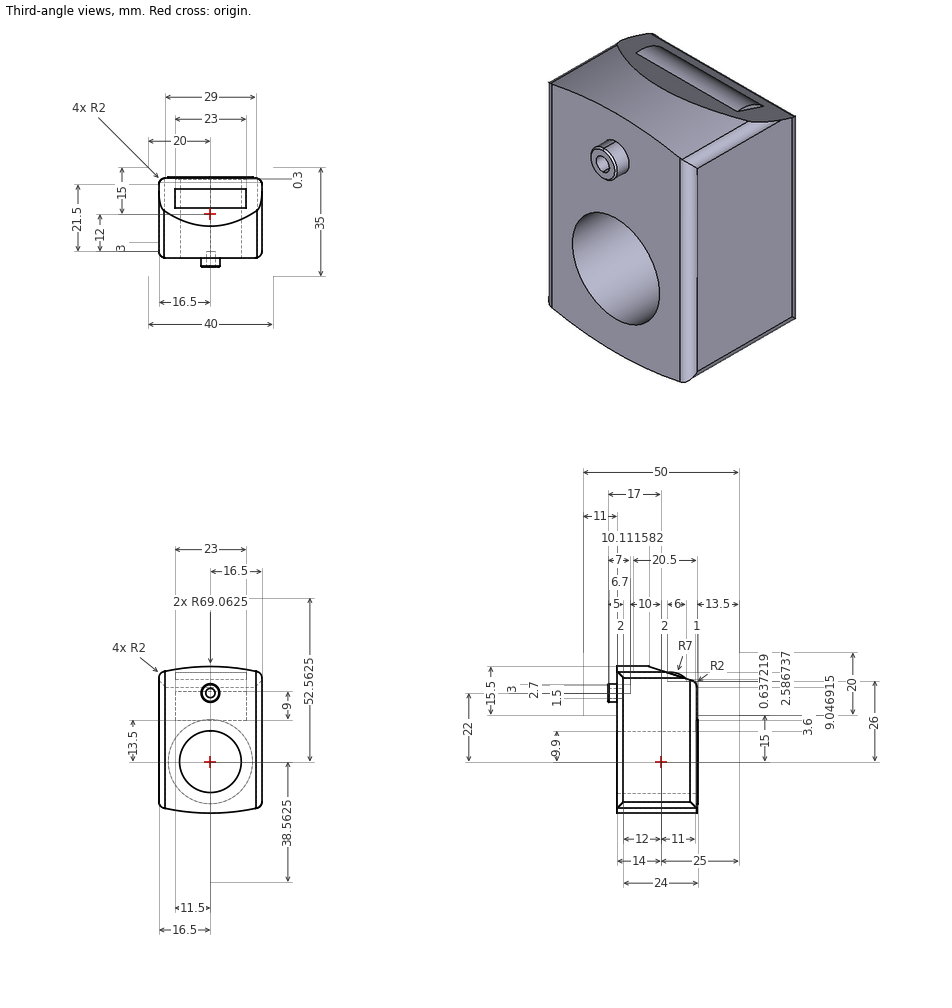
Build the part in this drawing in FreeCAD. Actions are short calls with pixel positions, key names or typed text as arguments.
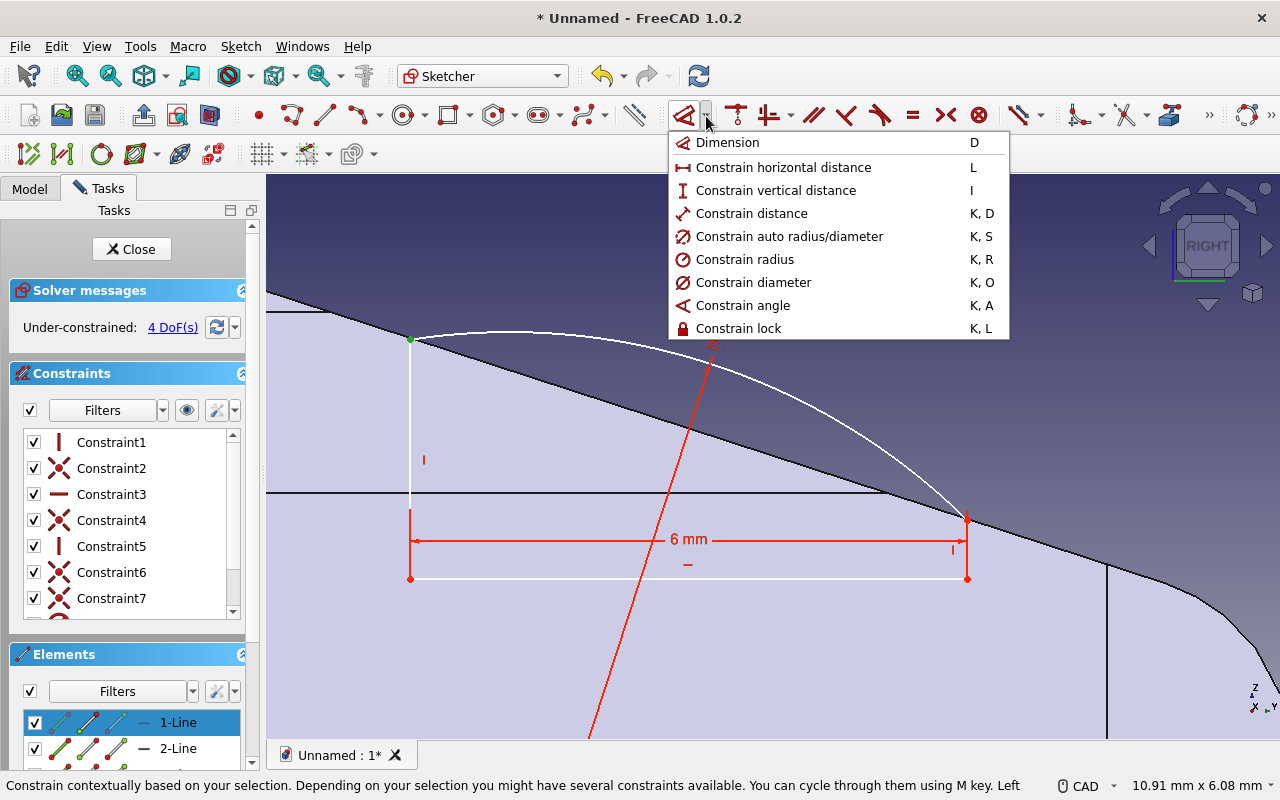
click(839, 168)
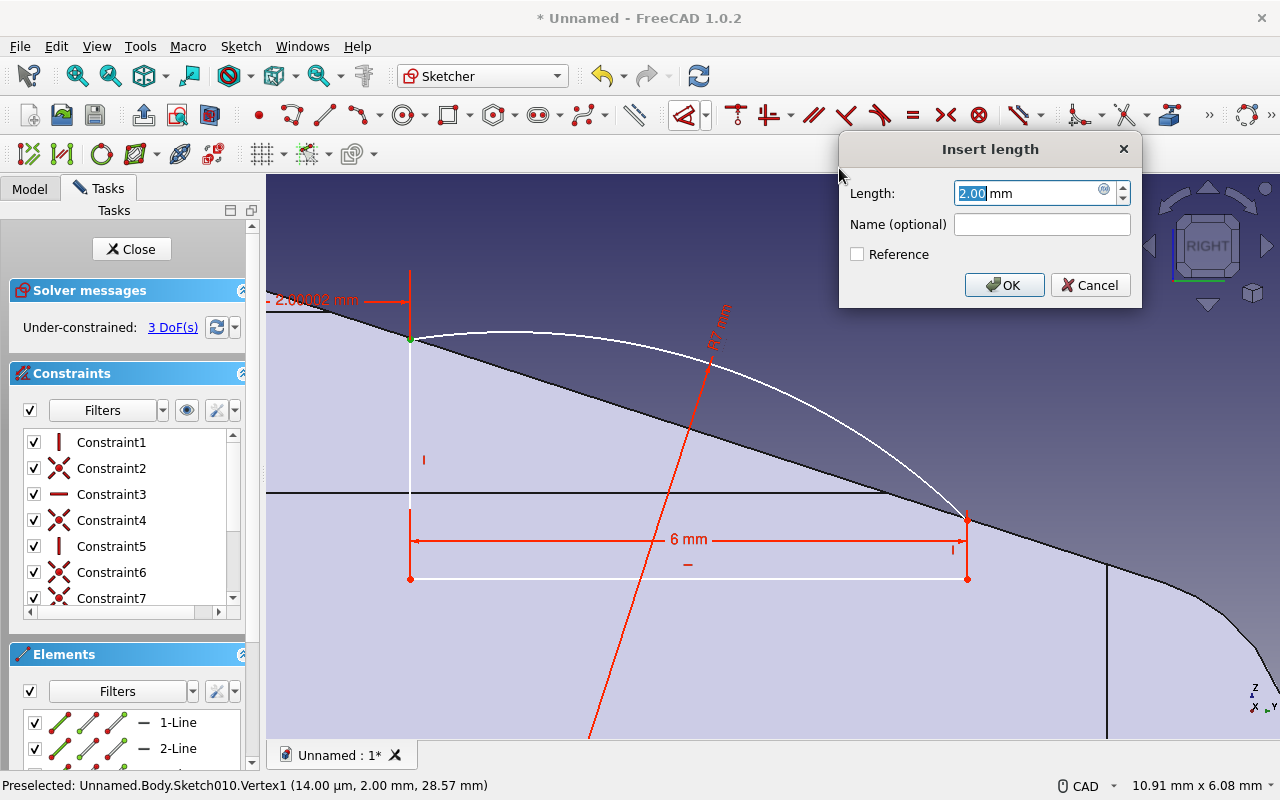
text(2)
key(Return)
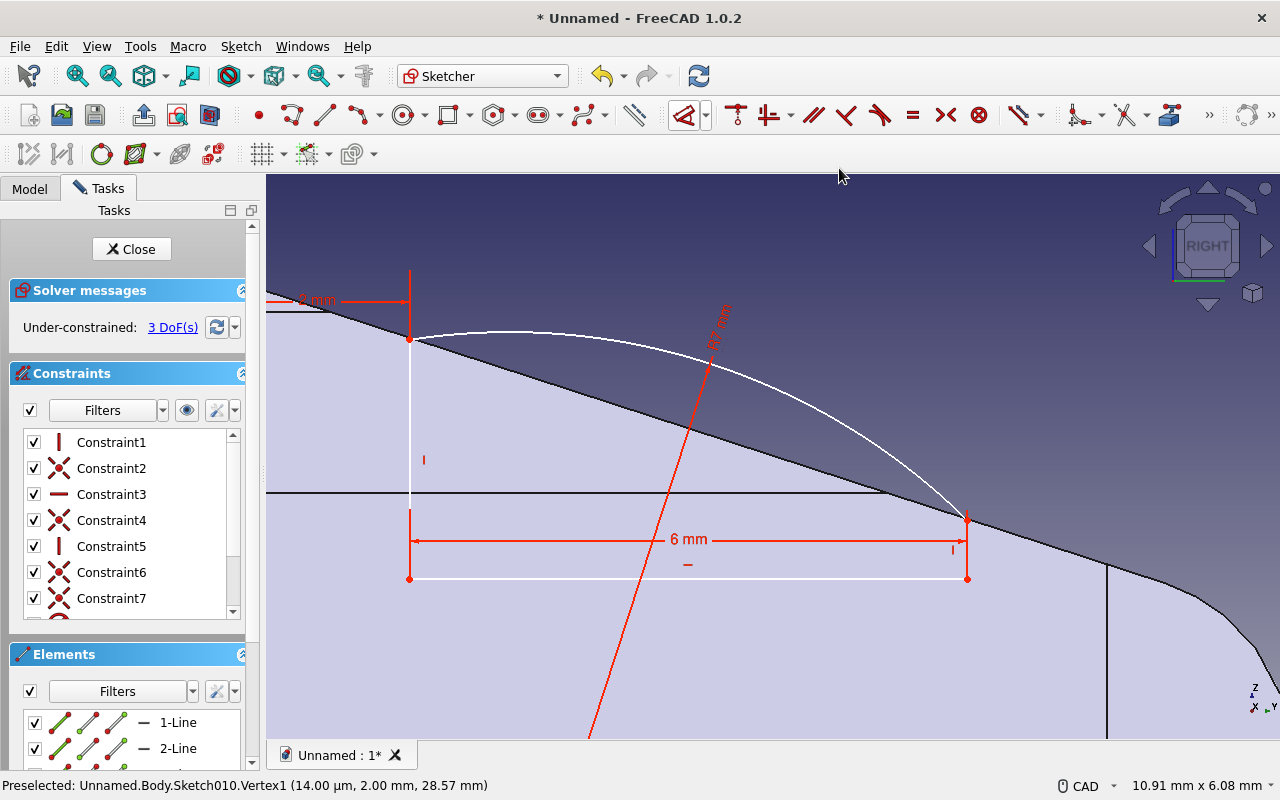
click(410, 579)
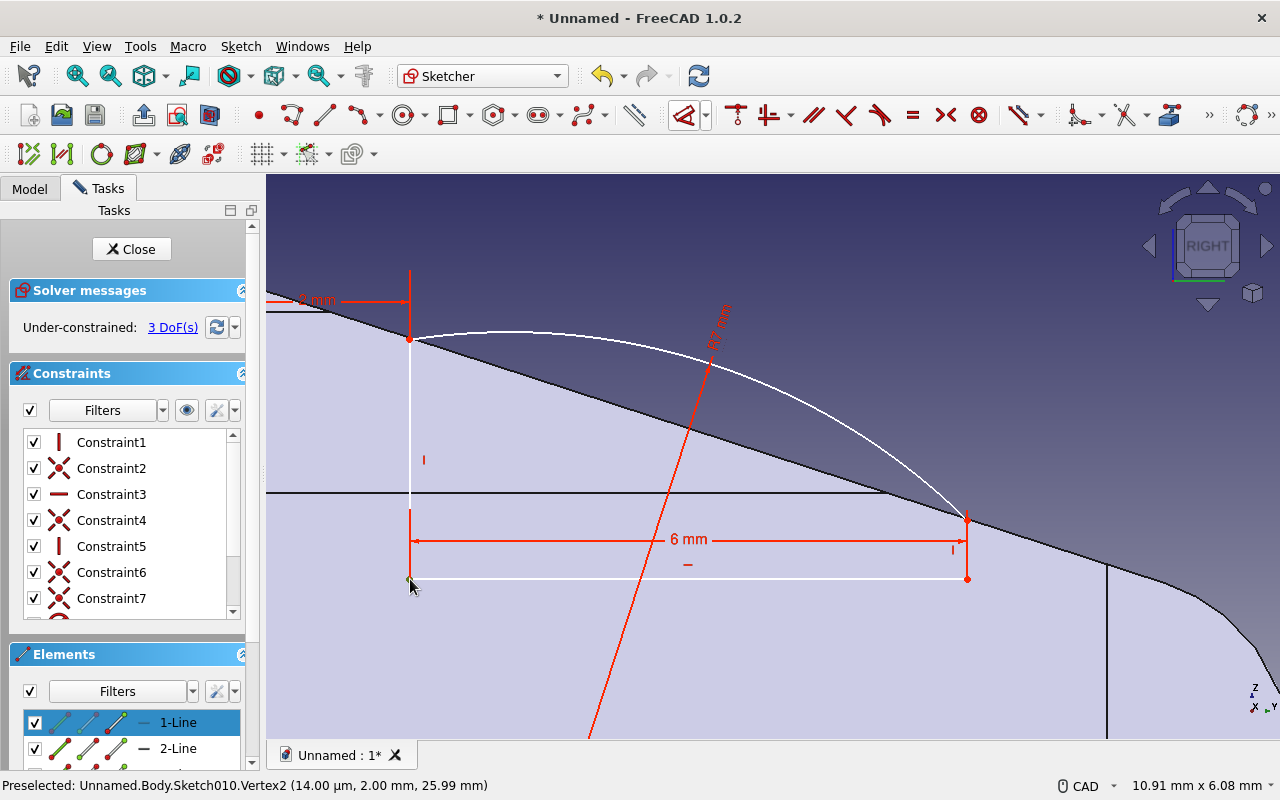
click(706, 116)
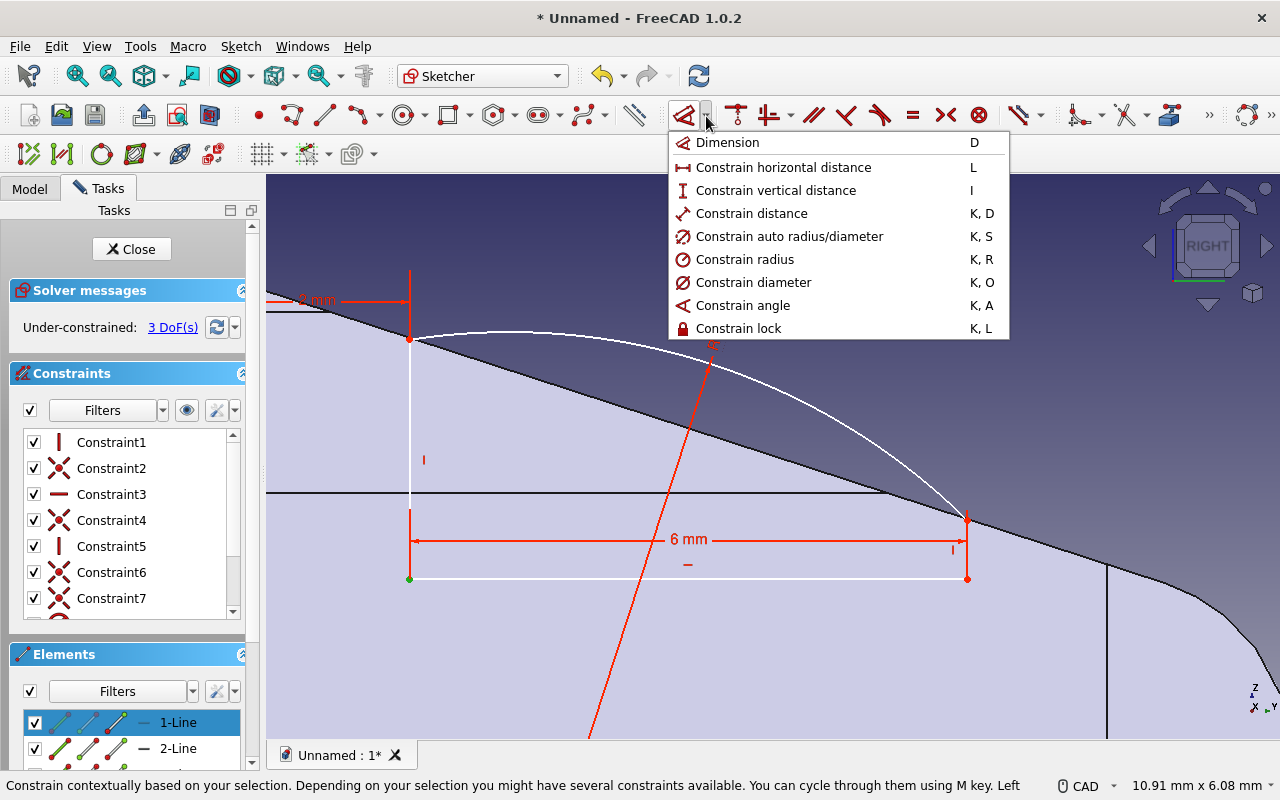
click(839, 190)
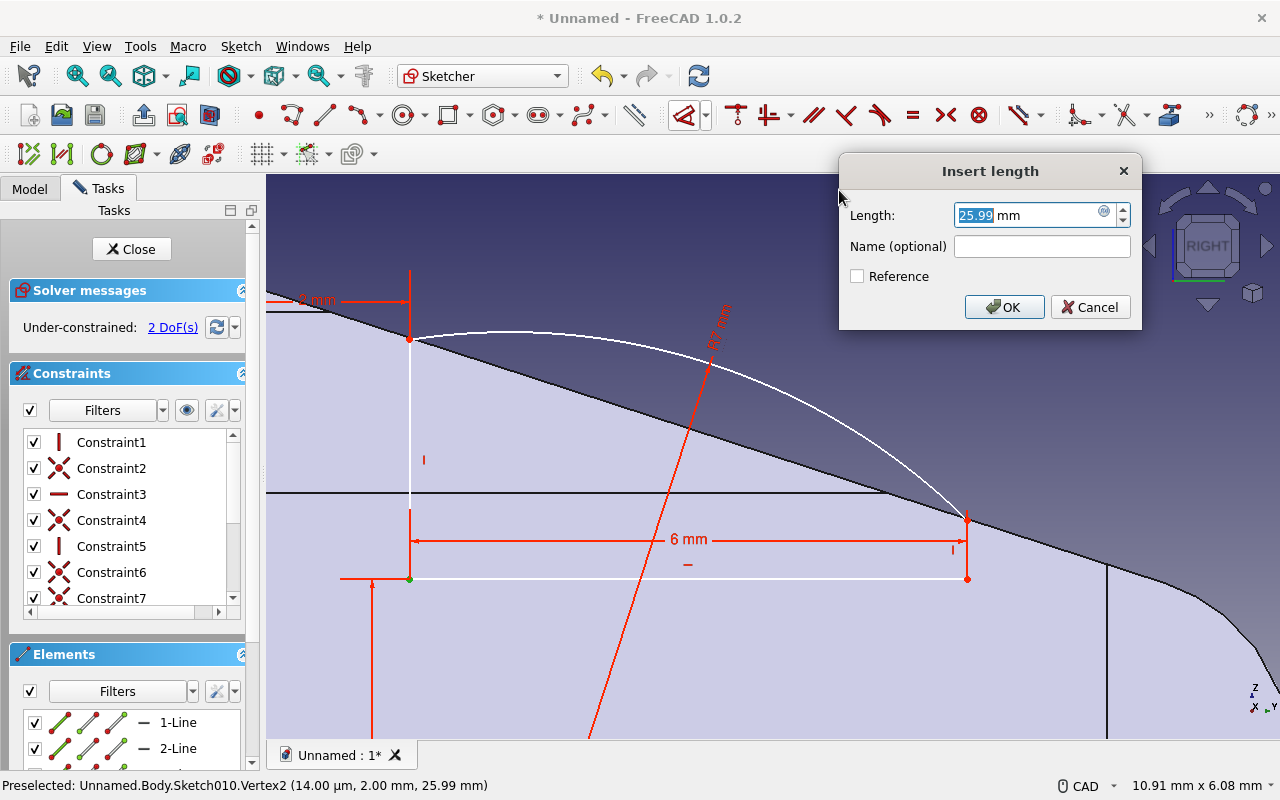
text(26)
key(Return)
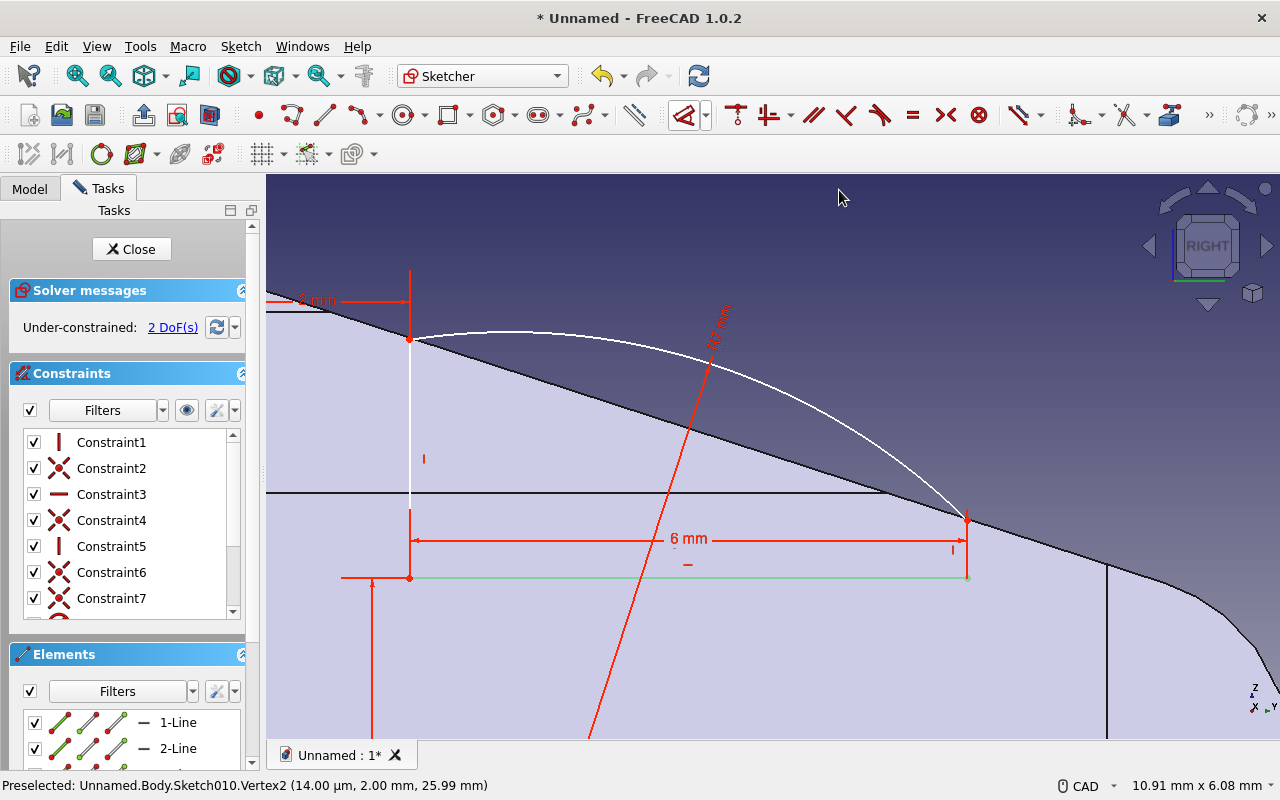
click(410, 411)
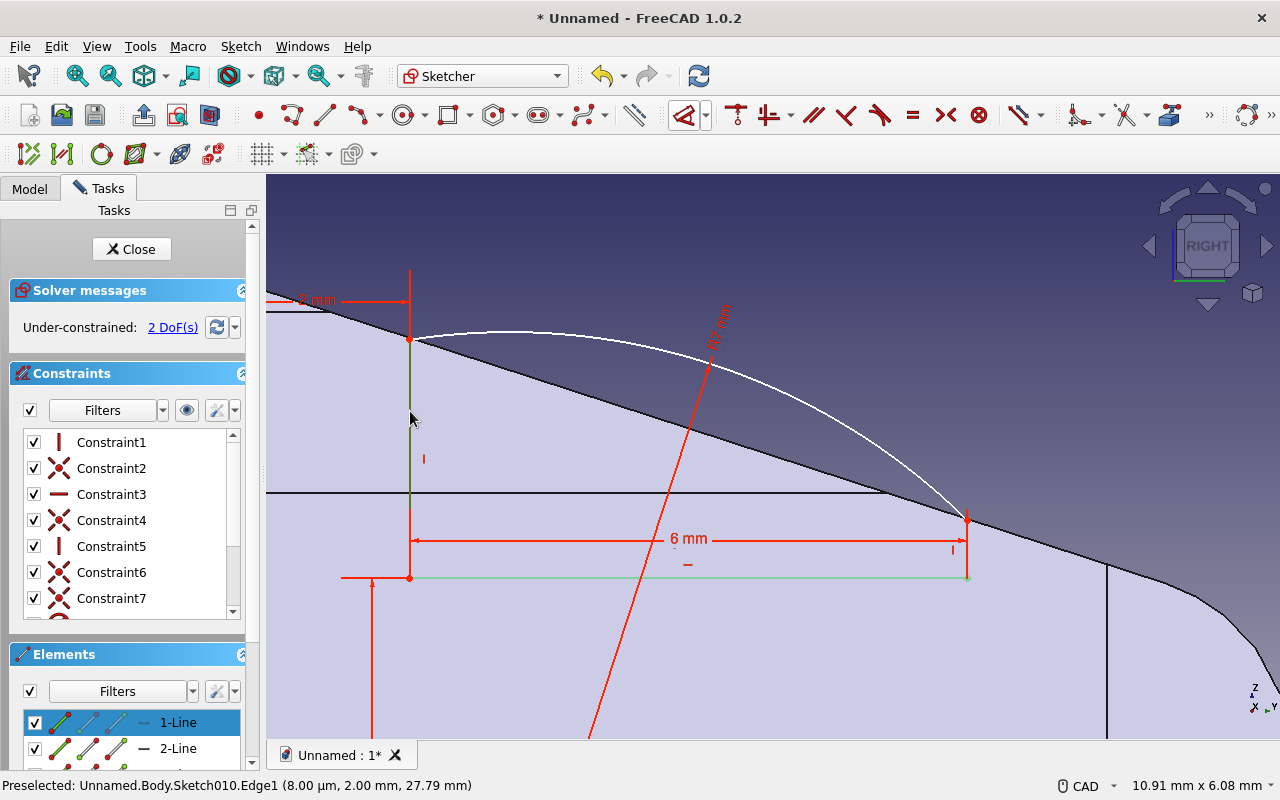
click(706, 116)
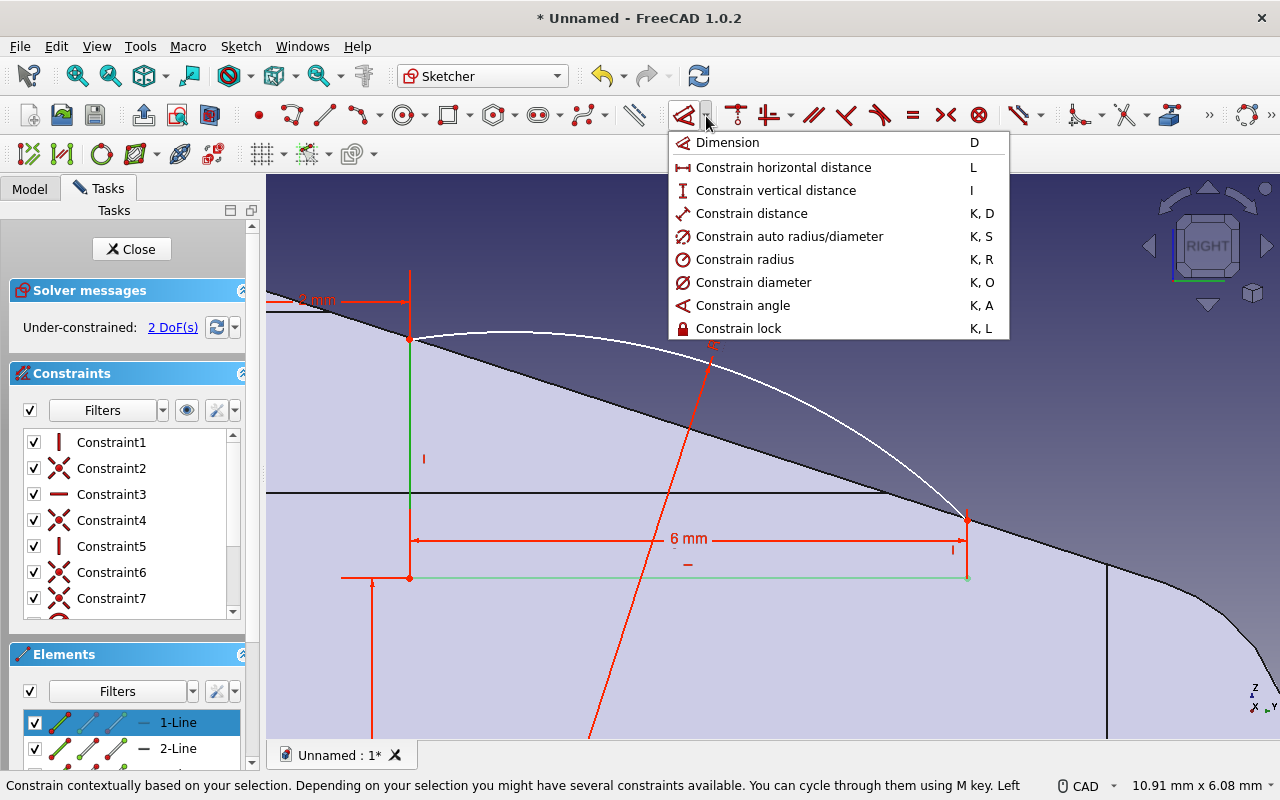
click(839, 190)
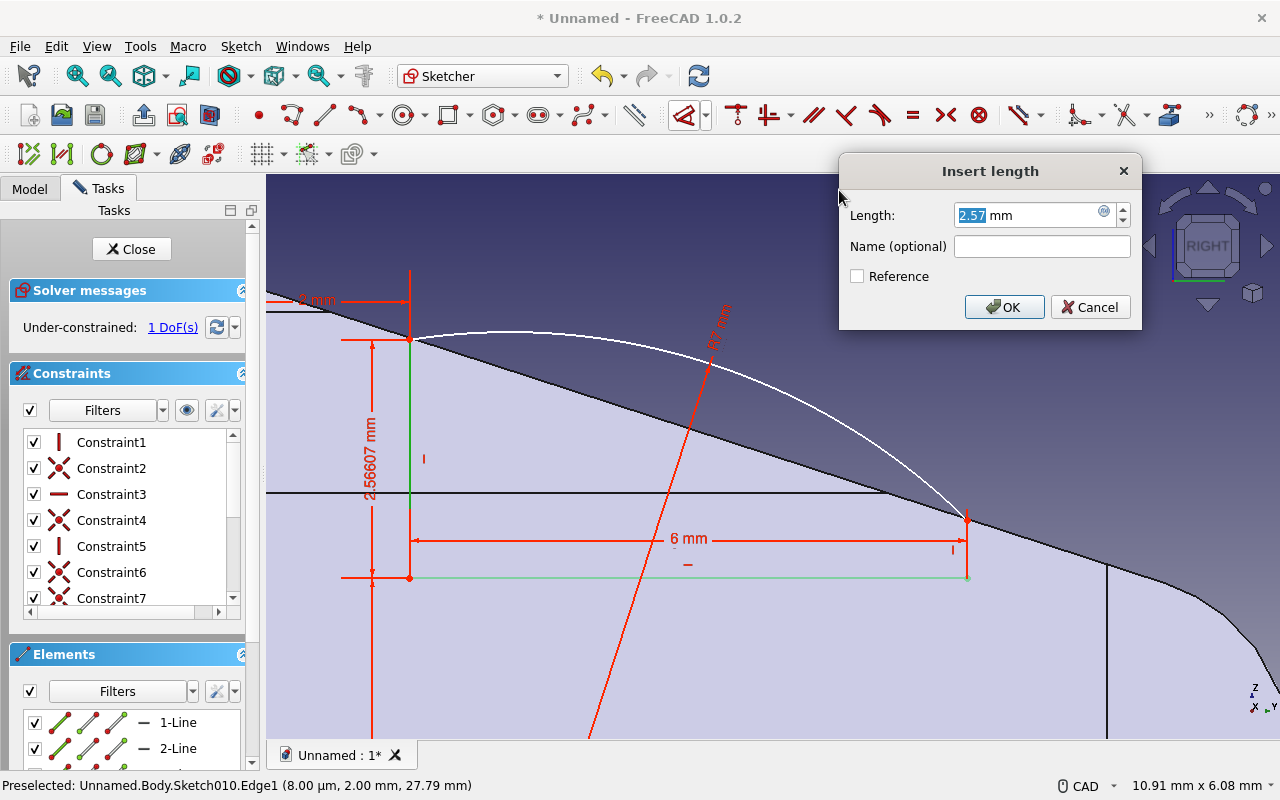
text(2.586737)
key(Return)